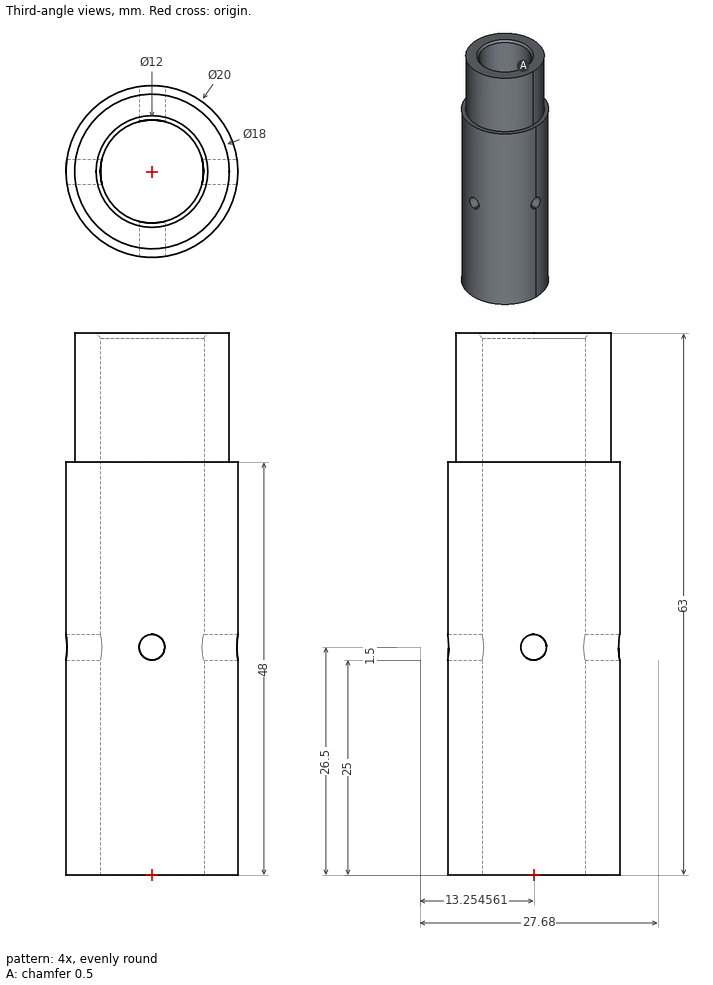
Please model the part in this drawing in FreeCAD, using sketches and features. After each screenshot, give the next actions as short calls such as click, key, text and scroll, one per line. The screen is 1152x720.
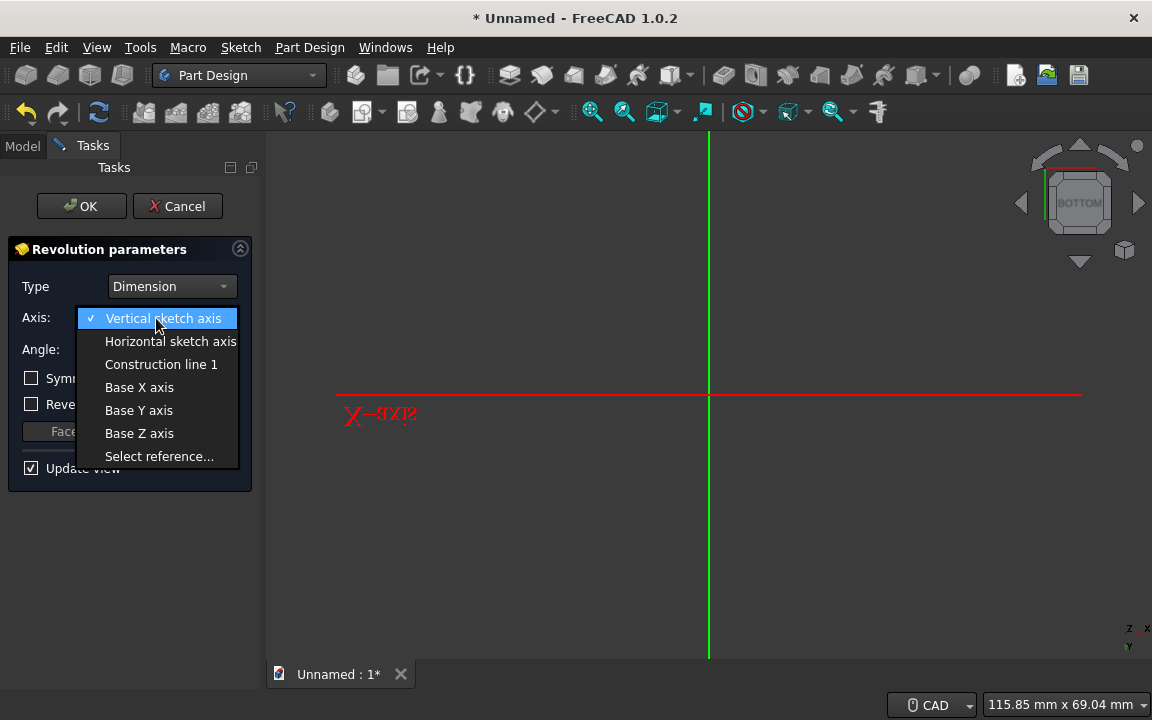
click(156, 364)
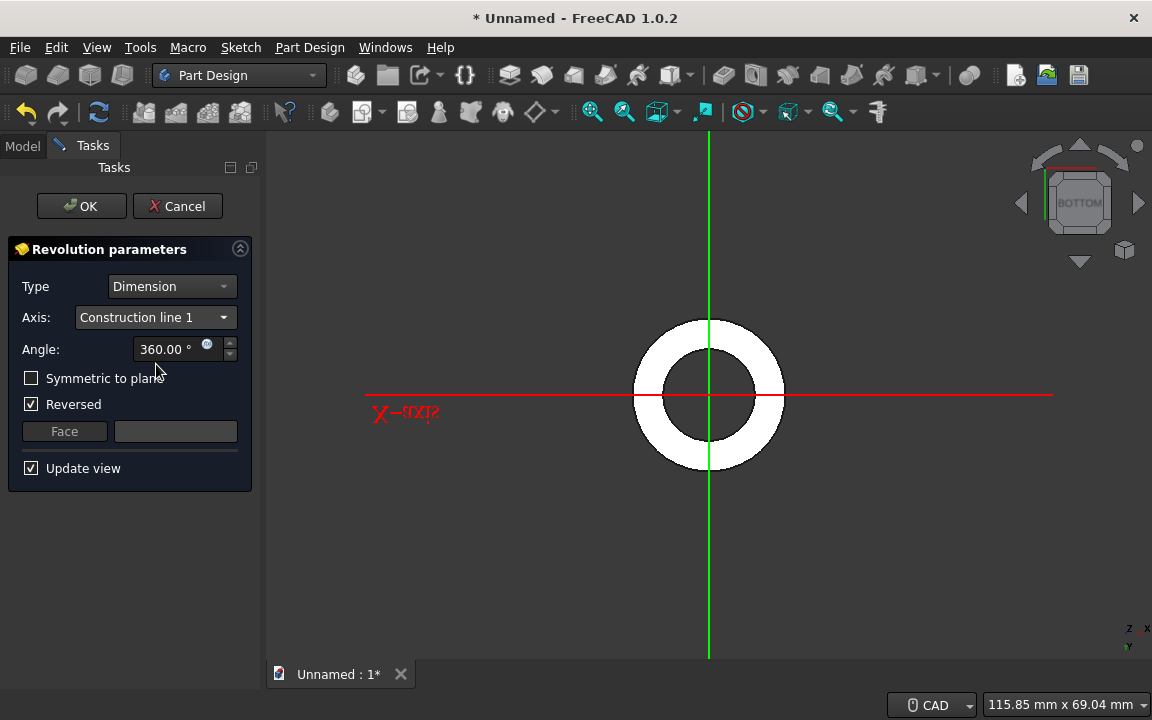
click(82, 206)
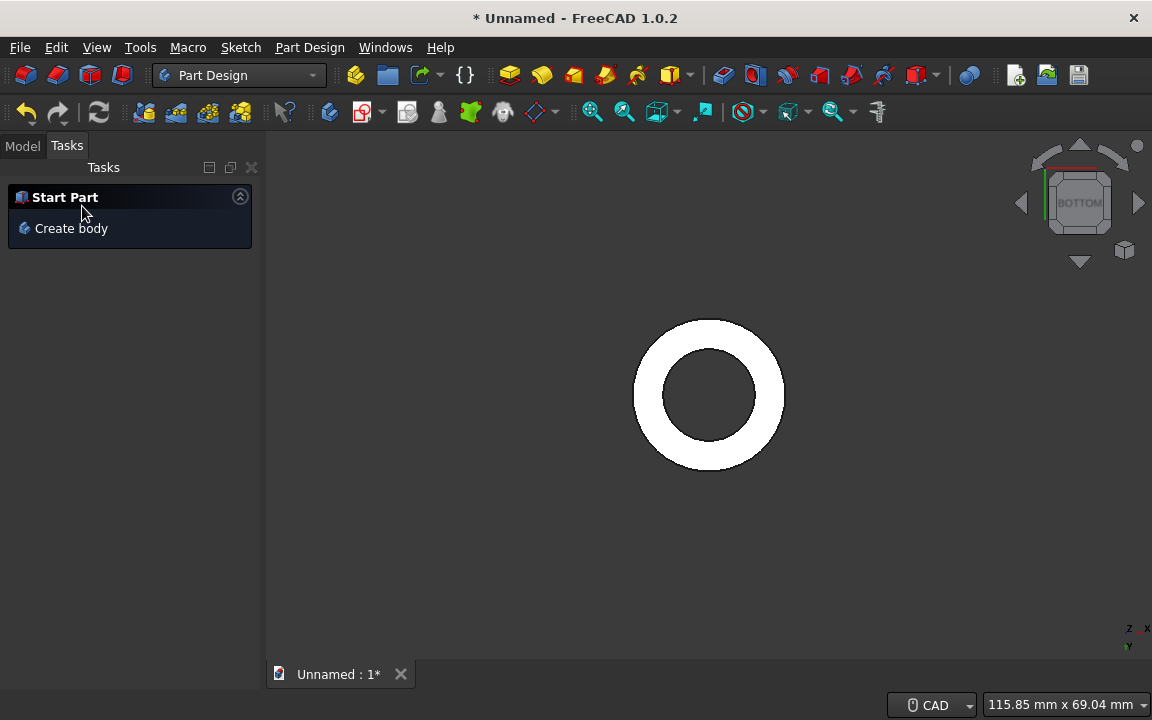
click(594, 112)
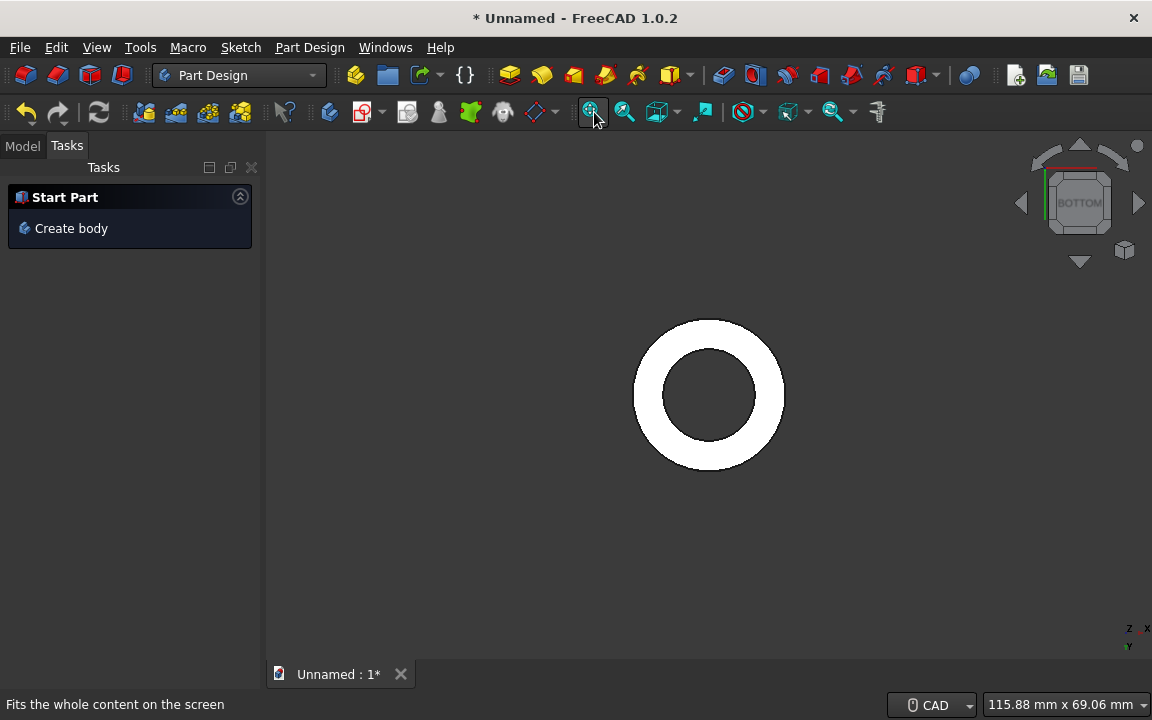
click(23, 145)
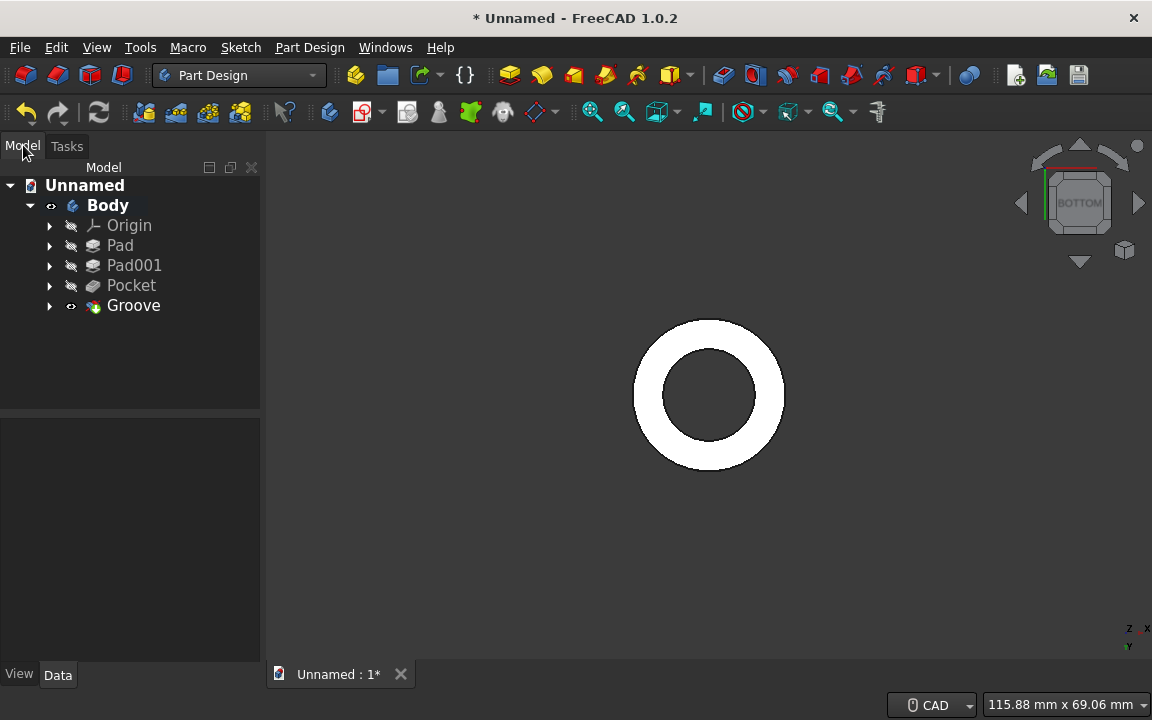
click(116, 306)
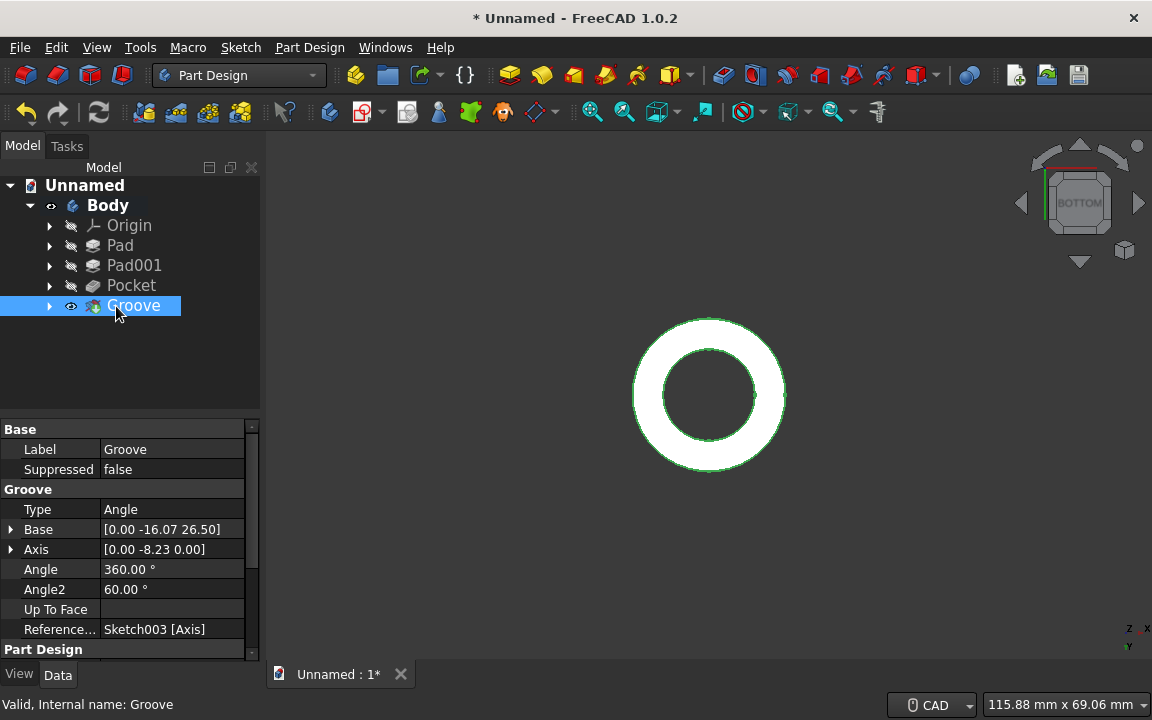
click(208, 112)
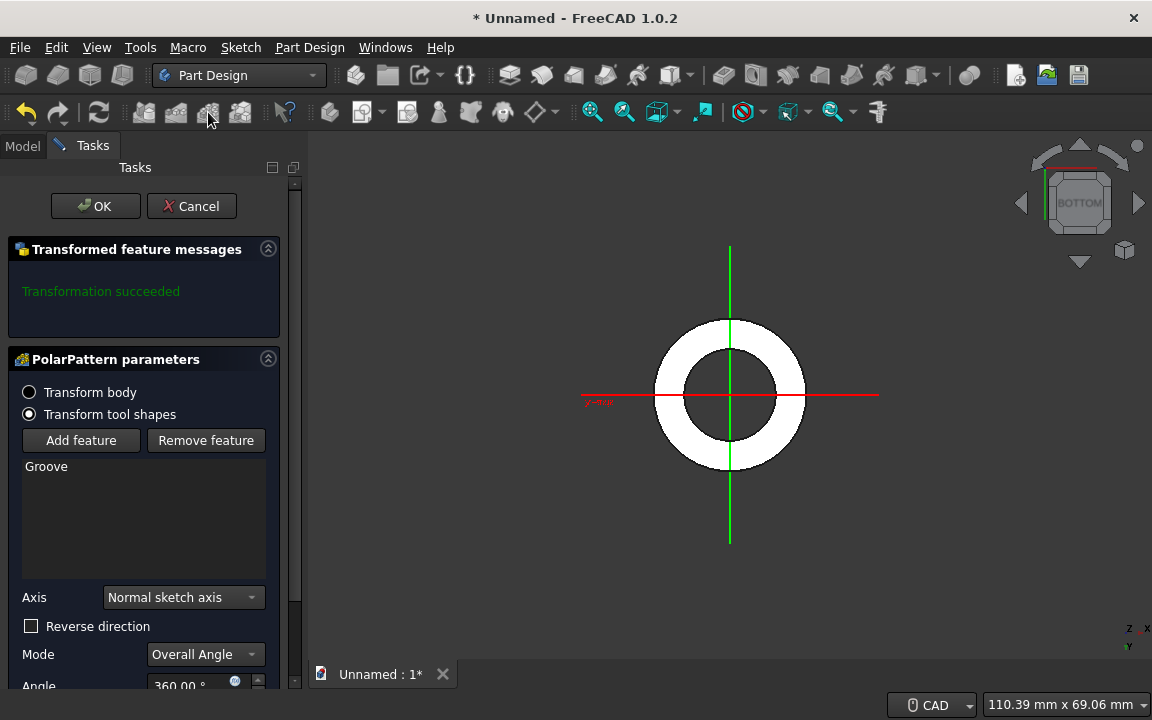
click(184, 598)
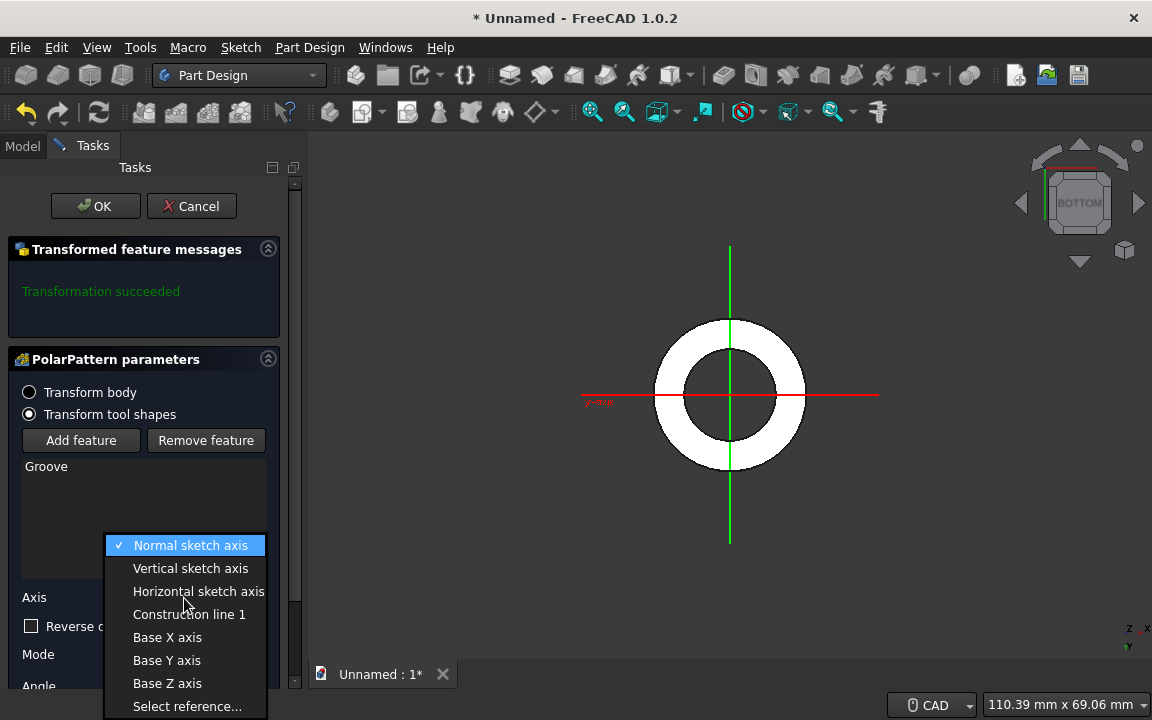
click(184, 684)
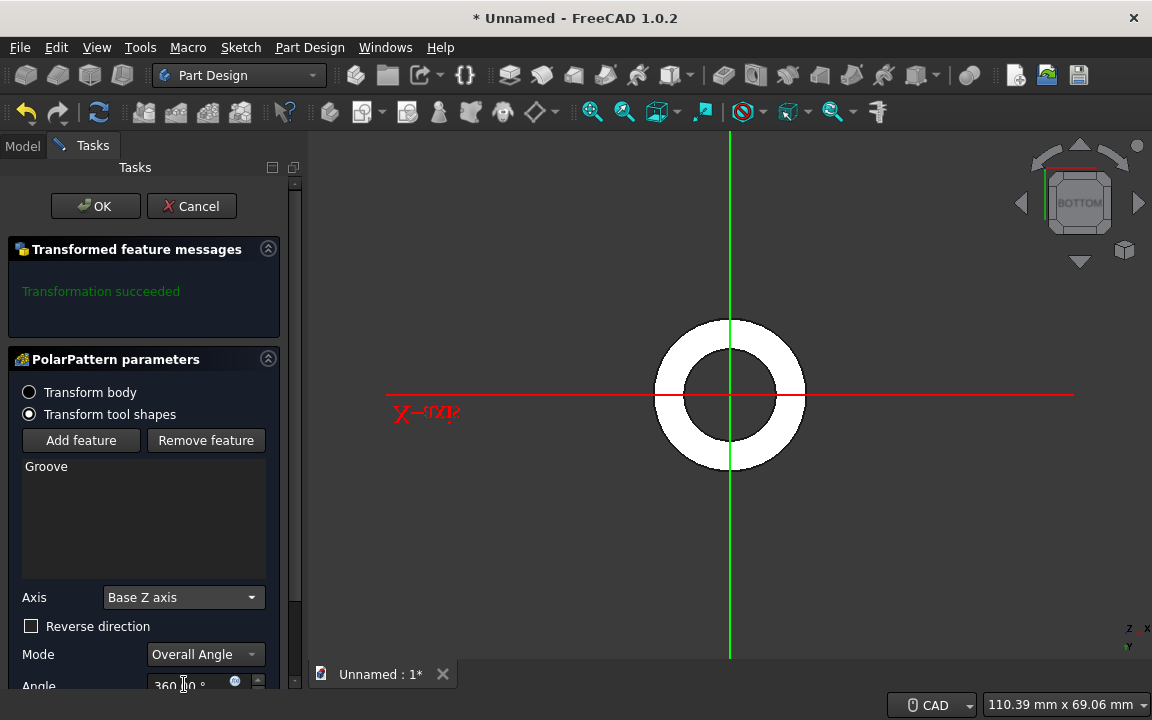
scroll(295, 432, down, 2)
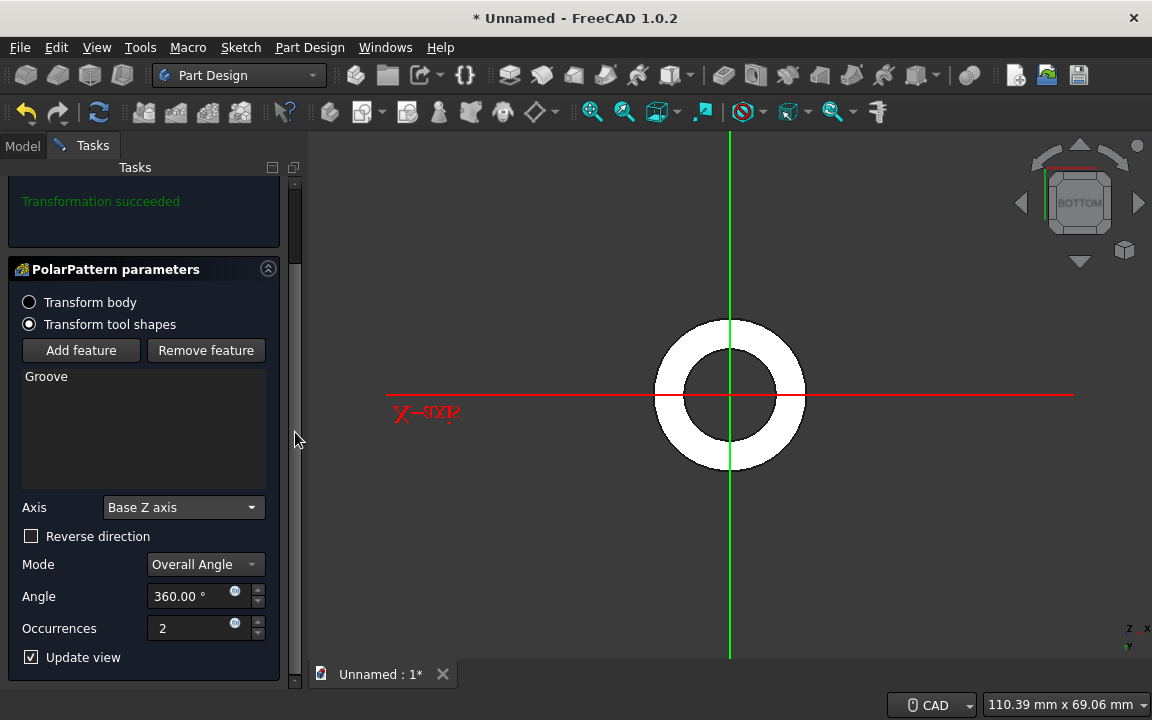
triple_click(198, 628)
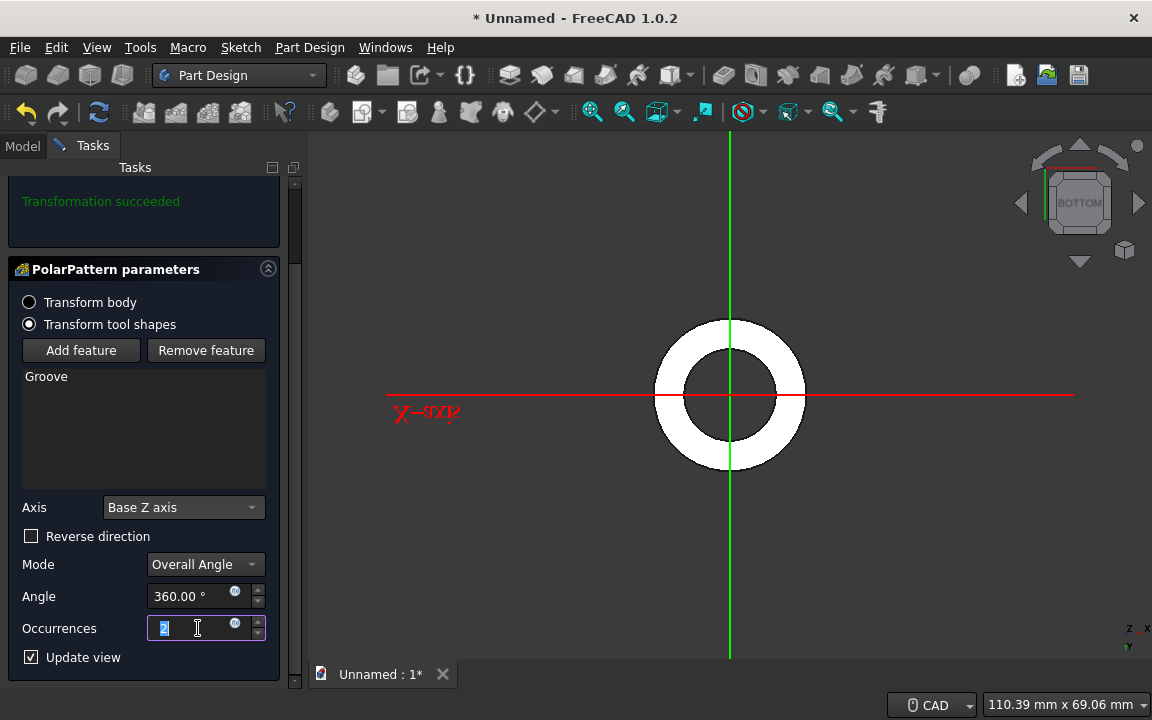
text(4)
key(Tab)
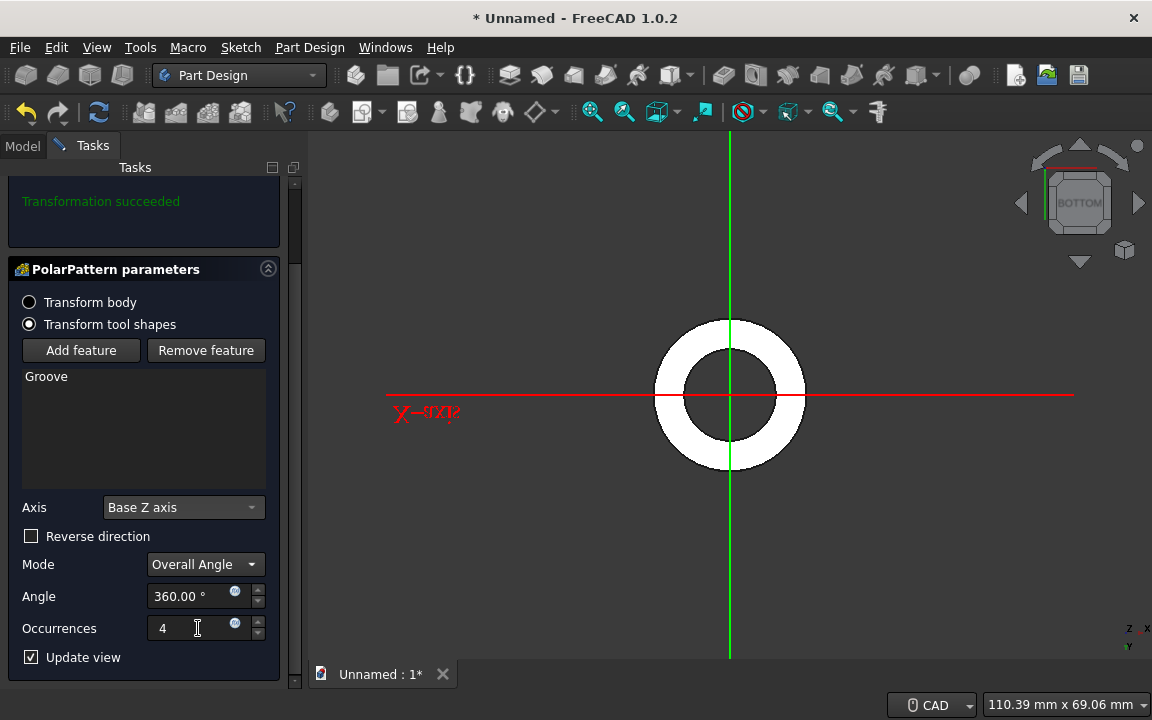
scroll(295, 432, up, 3)